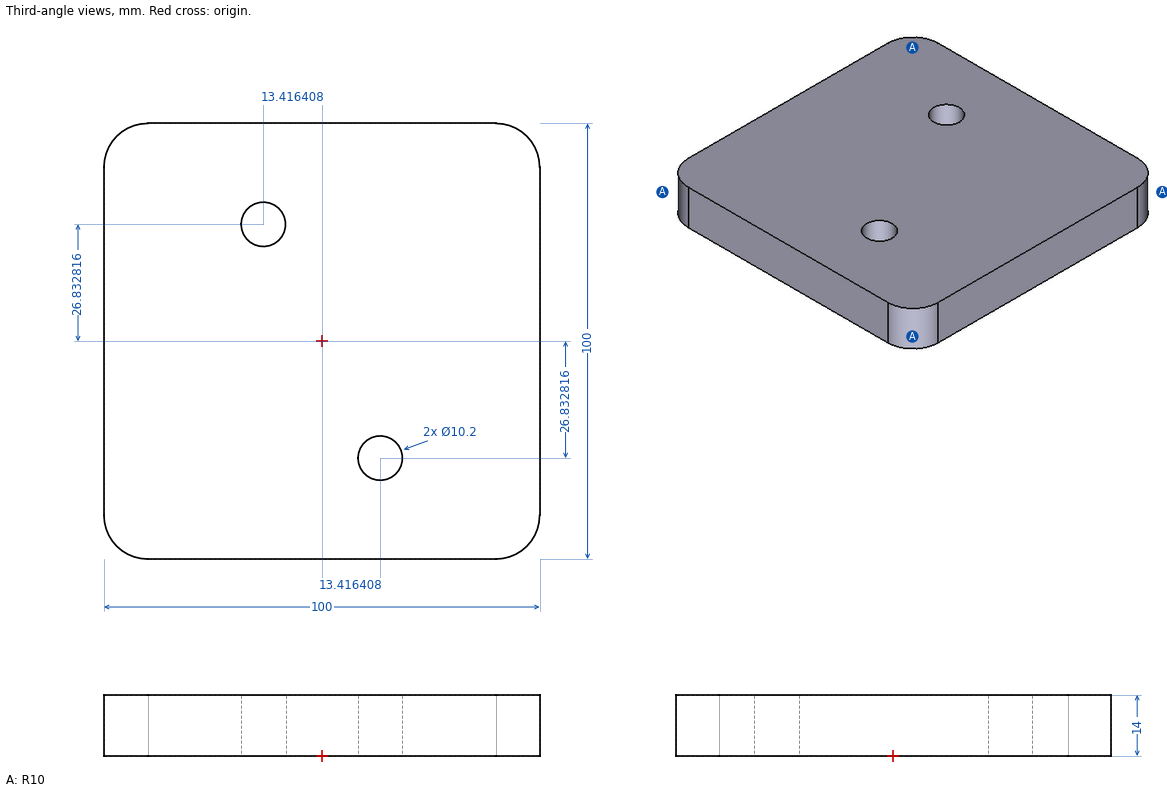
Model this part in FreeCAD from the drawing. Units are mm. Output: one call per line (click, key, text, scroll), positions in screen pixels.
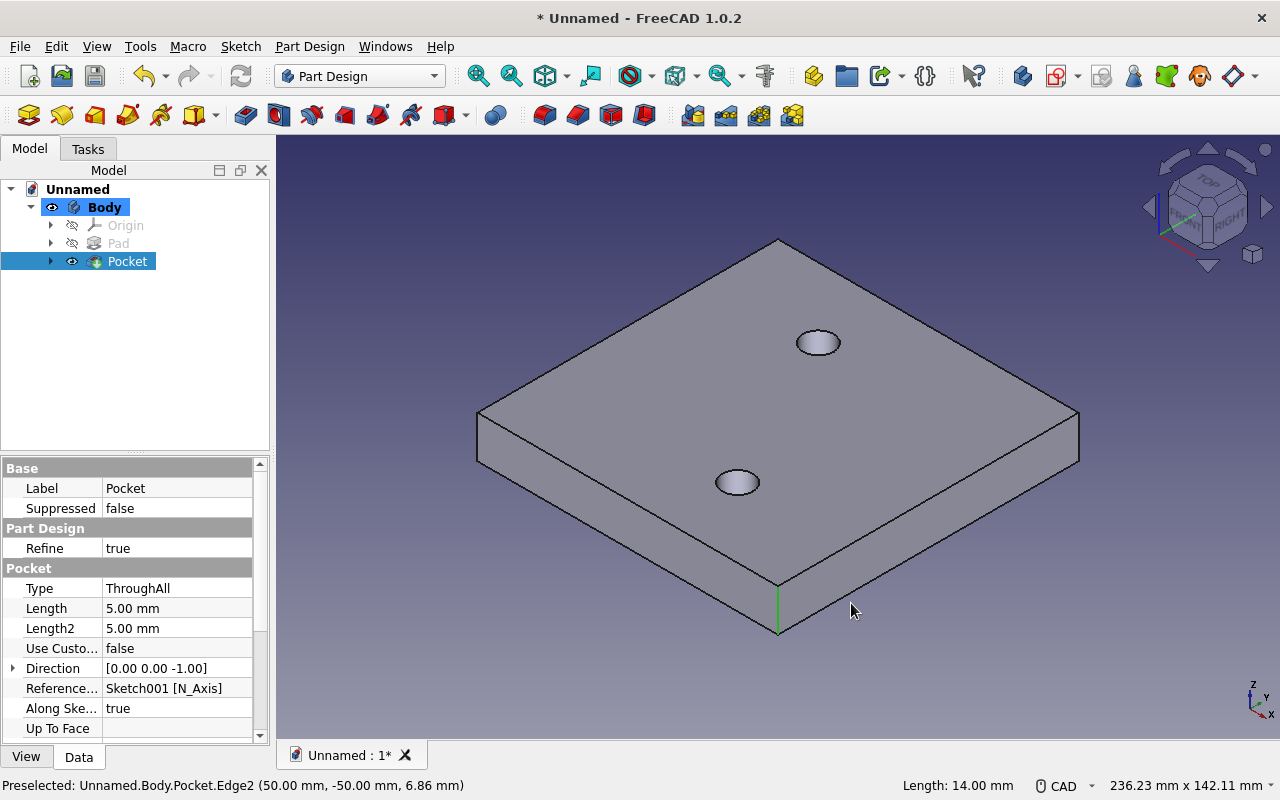
key(2)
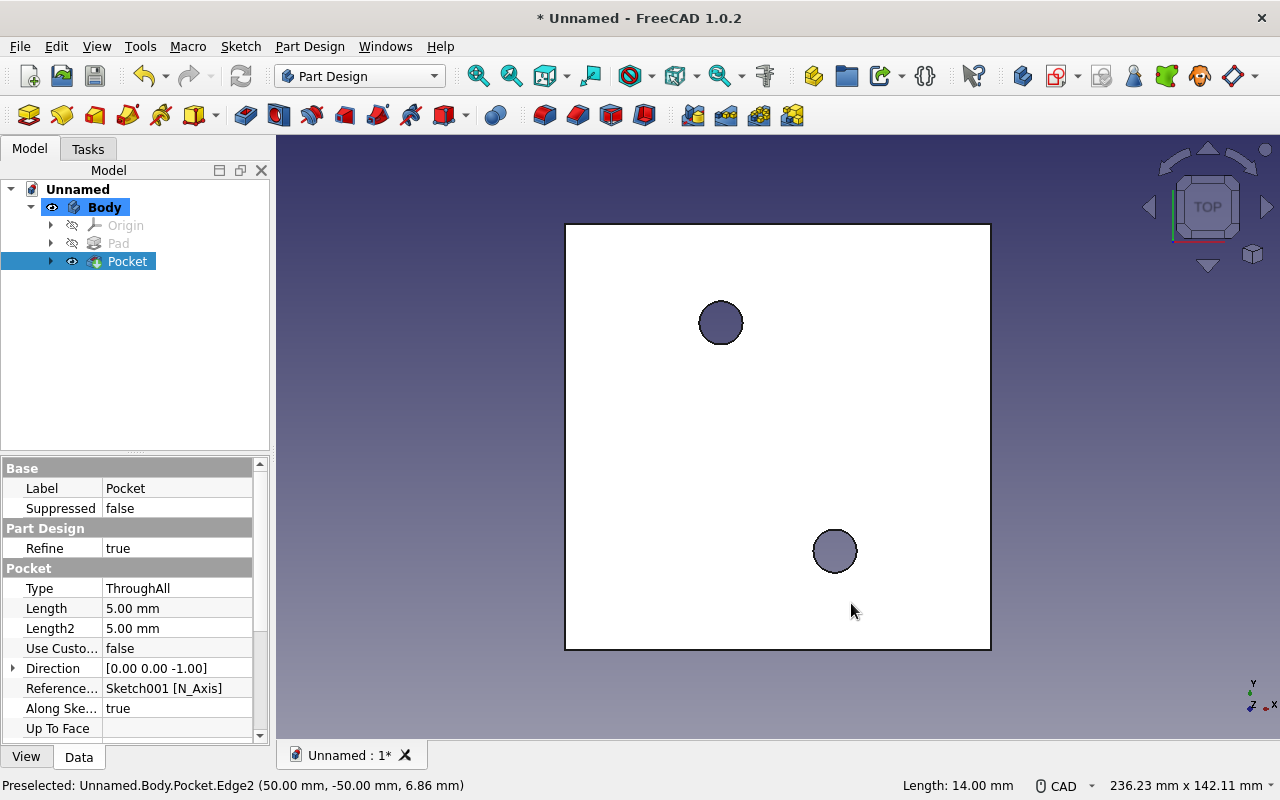
key(1)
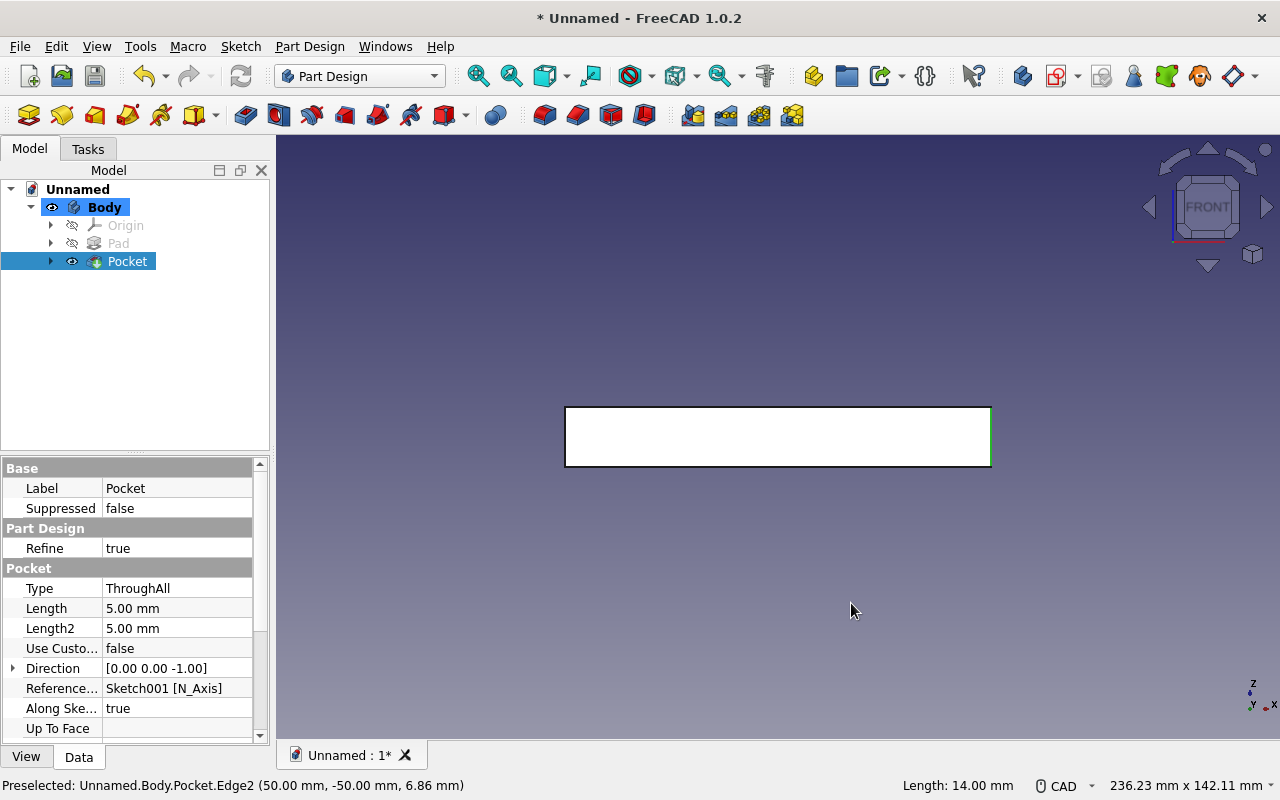
click(479, 76)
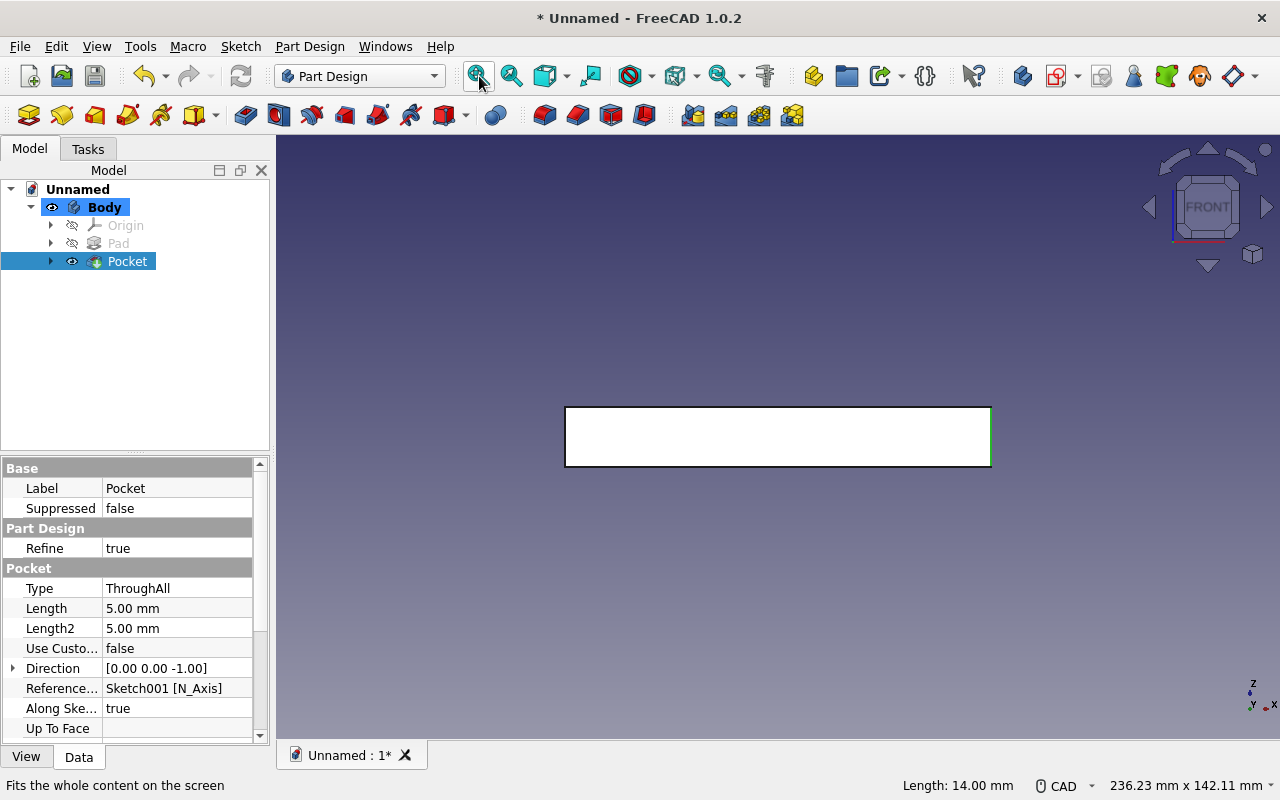
click(565, 436, ctrl)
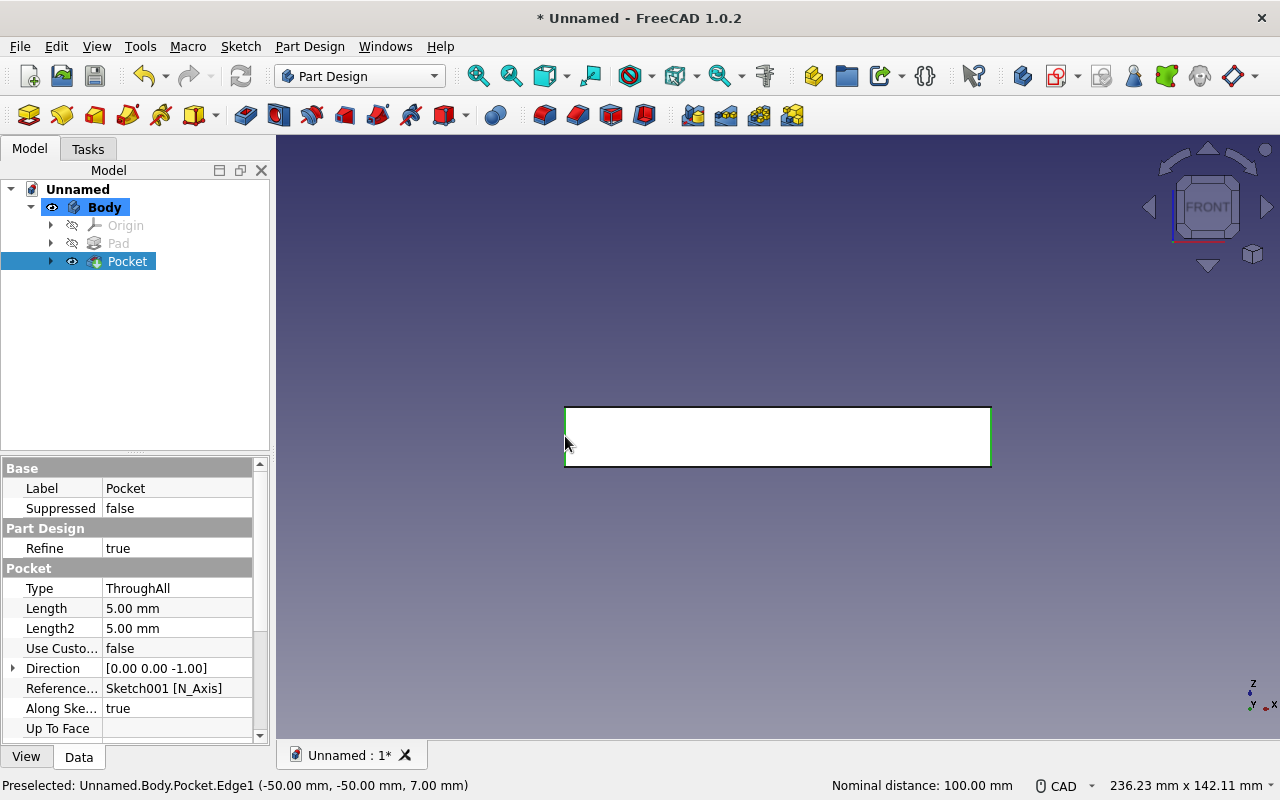
key(3)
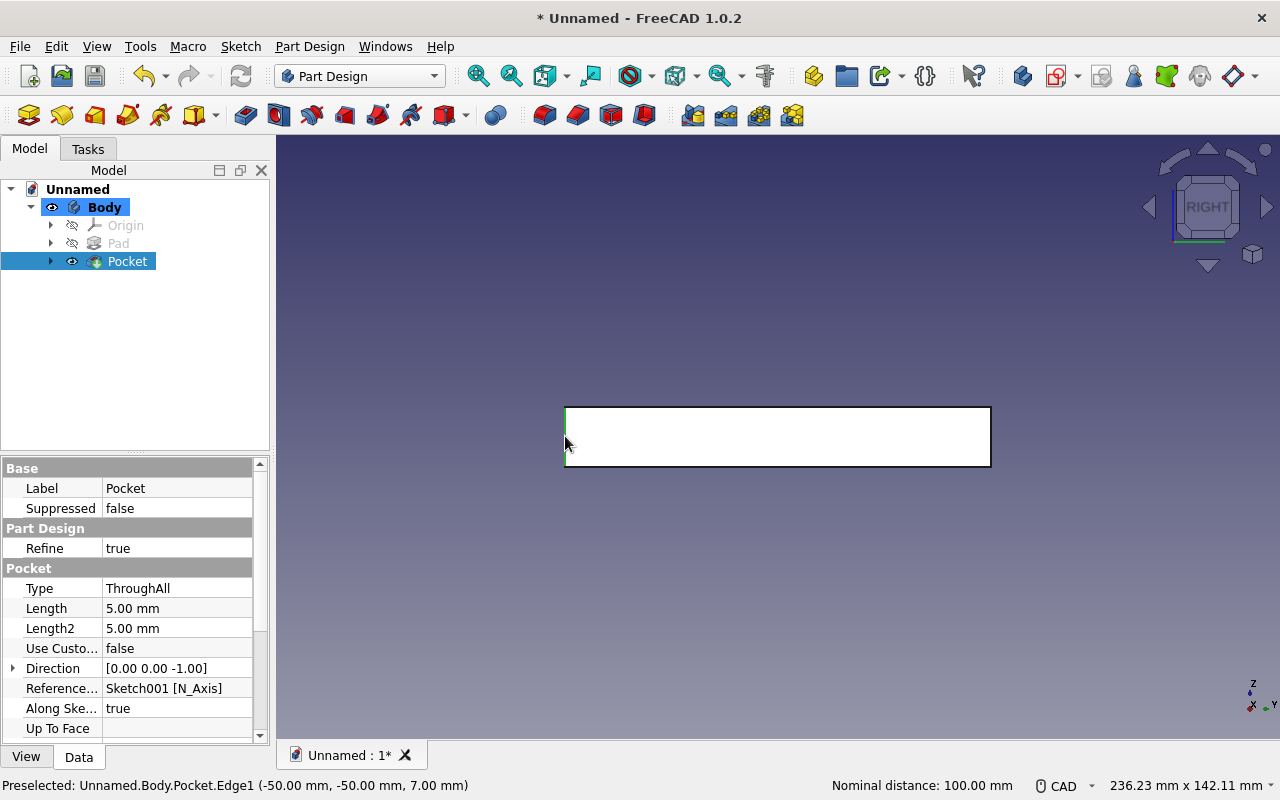
click(479, 76)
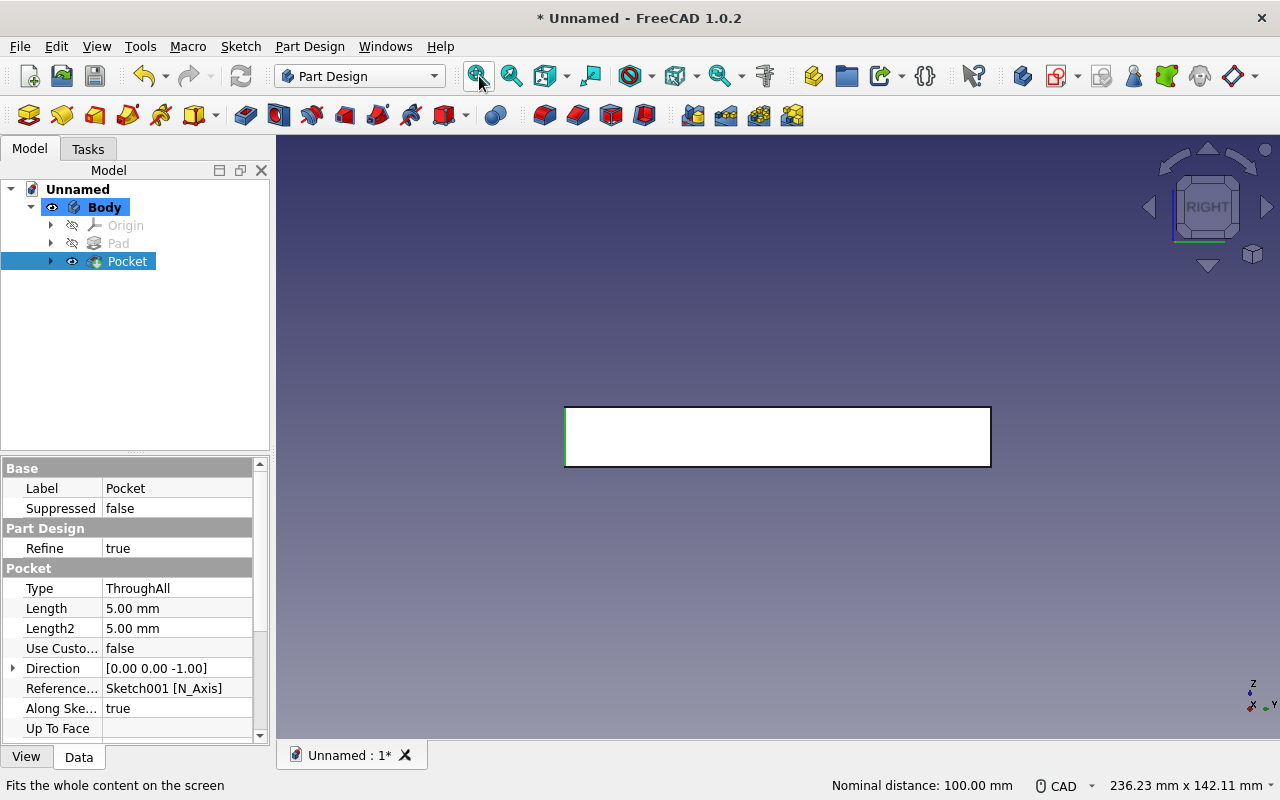
click(991, 436, ctrl)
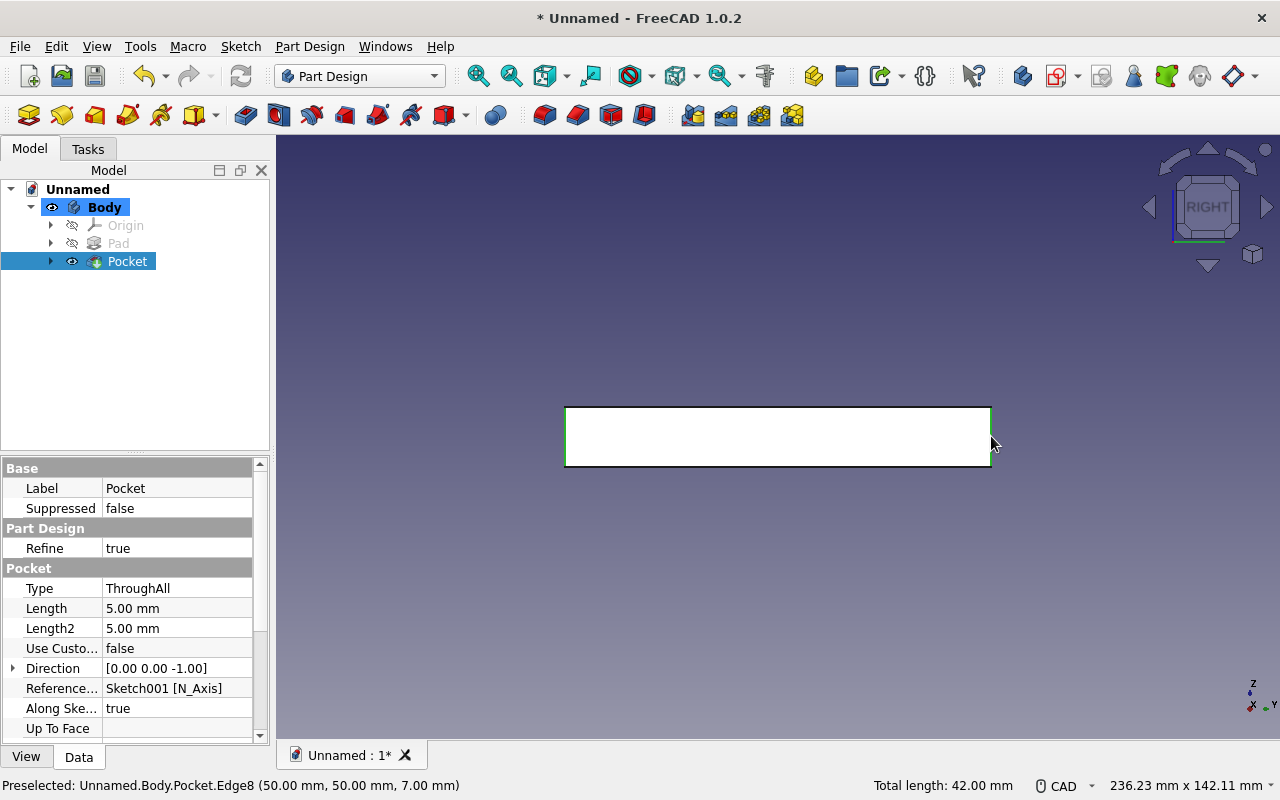
key(5)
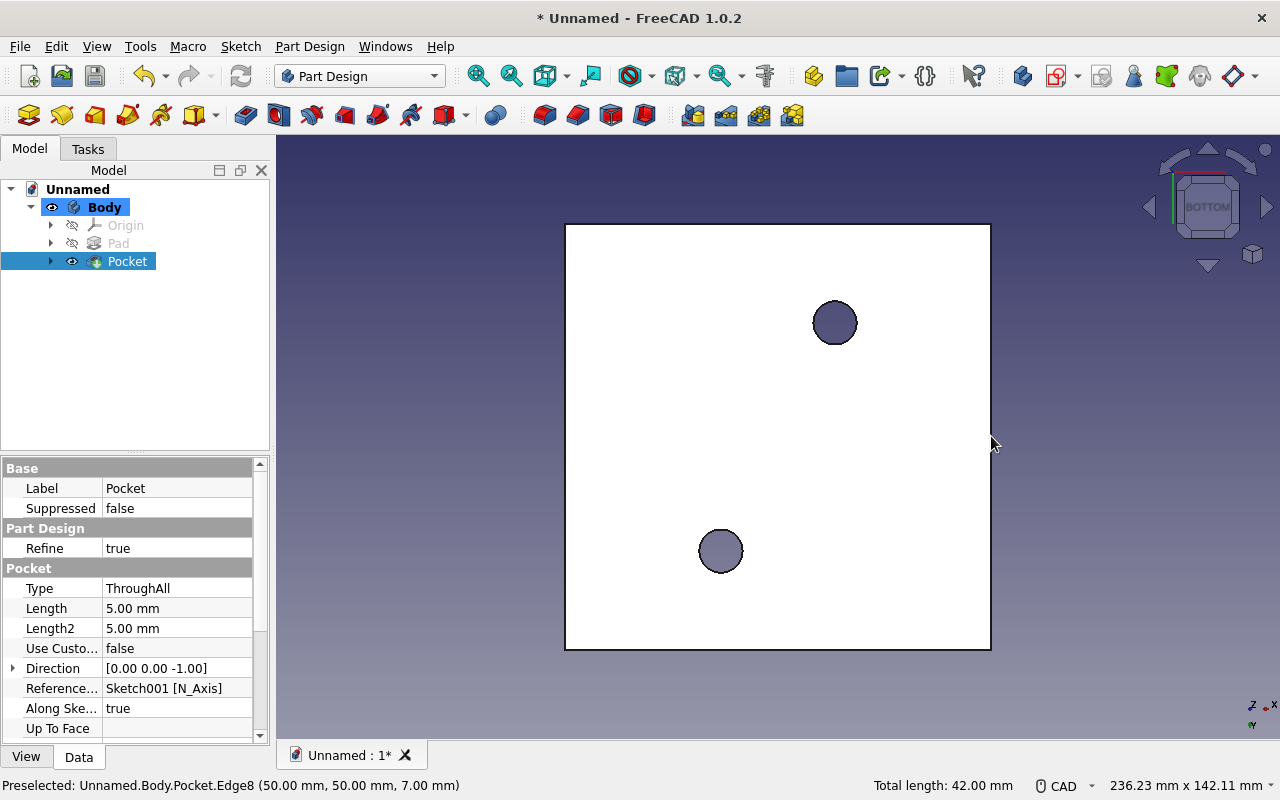
key(4)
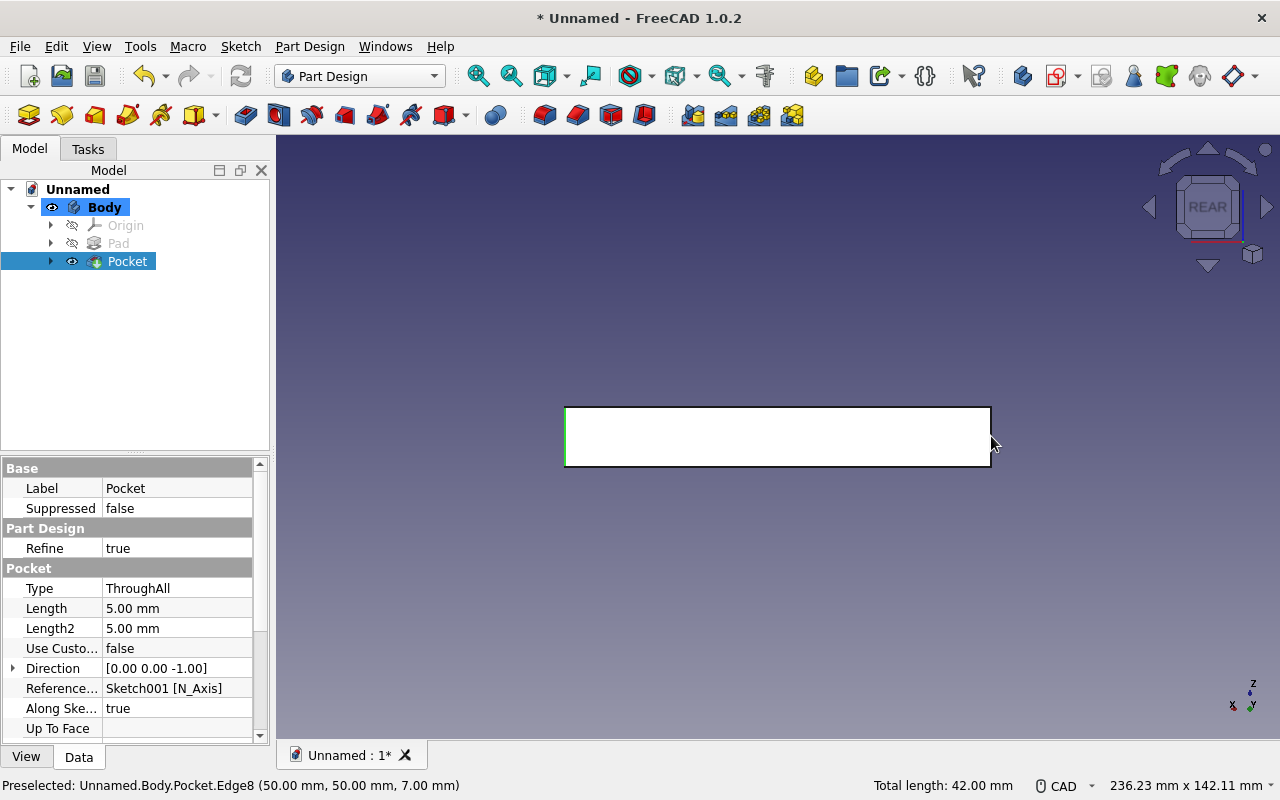
click(479, 76)